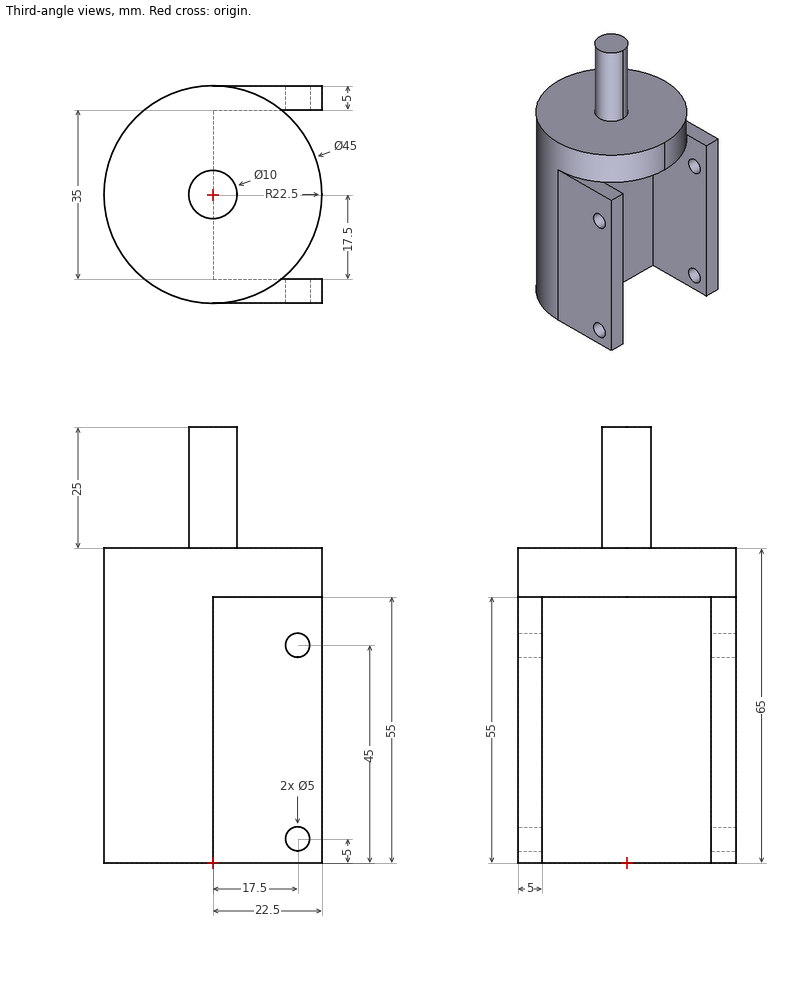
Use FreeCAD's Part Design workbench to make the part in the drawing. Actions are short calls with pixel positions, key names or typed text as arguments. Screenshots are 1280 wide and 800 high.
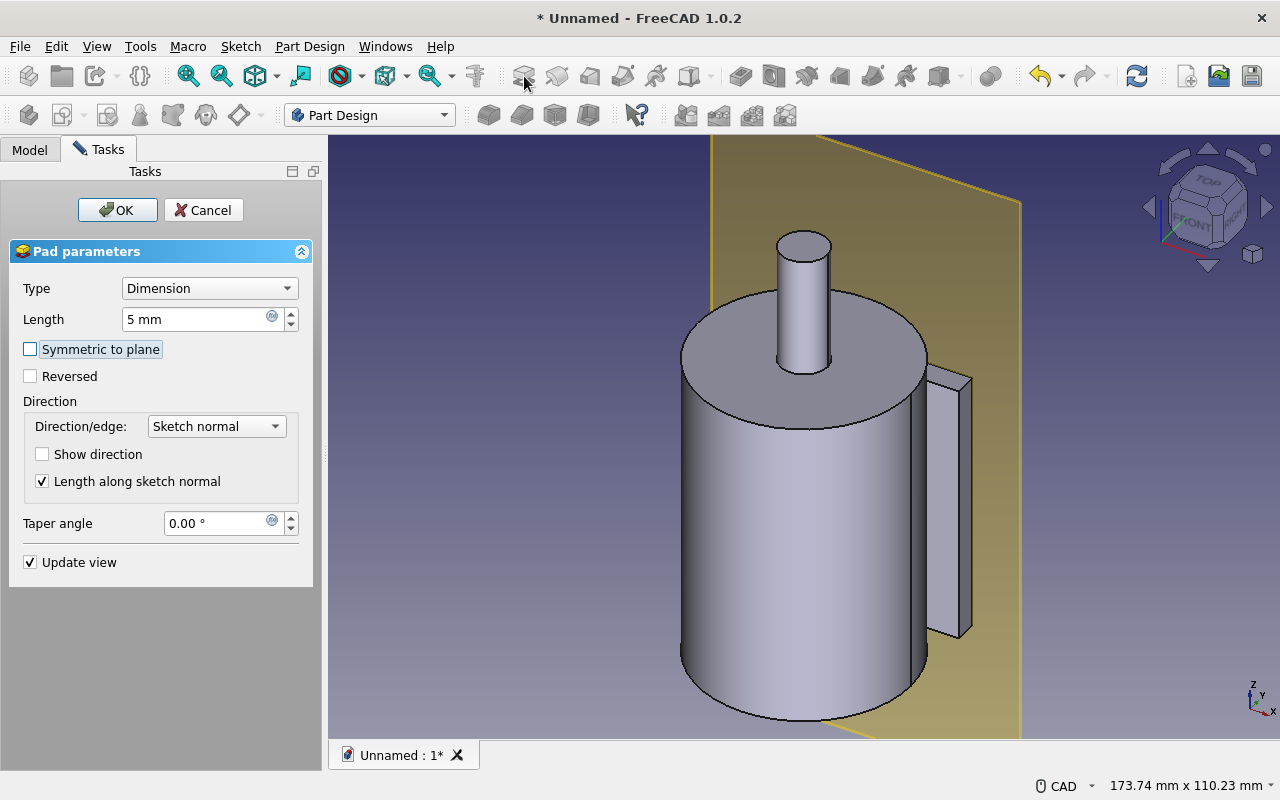
click(118, 210)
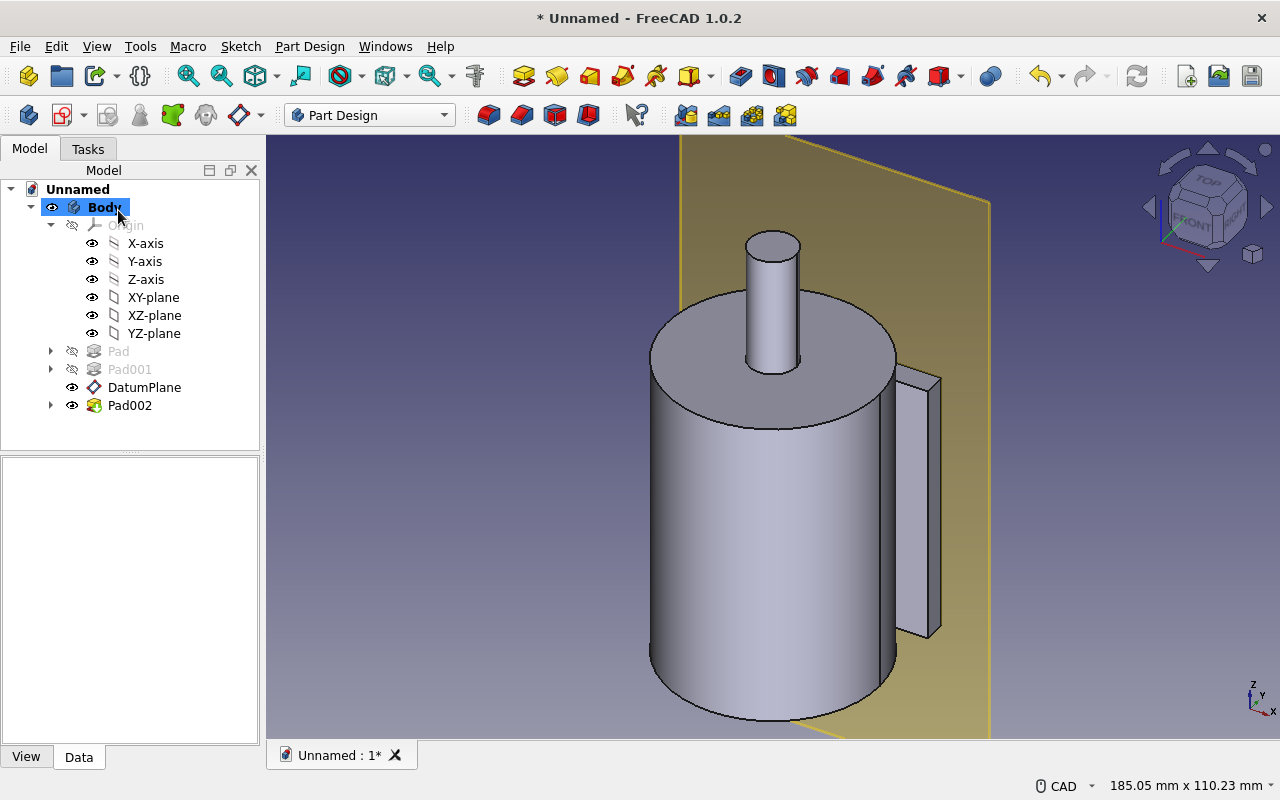
click(117, 387)
key(space)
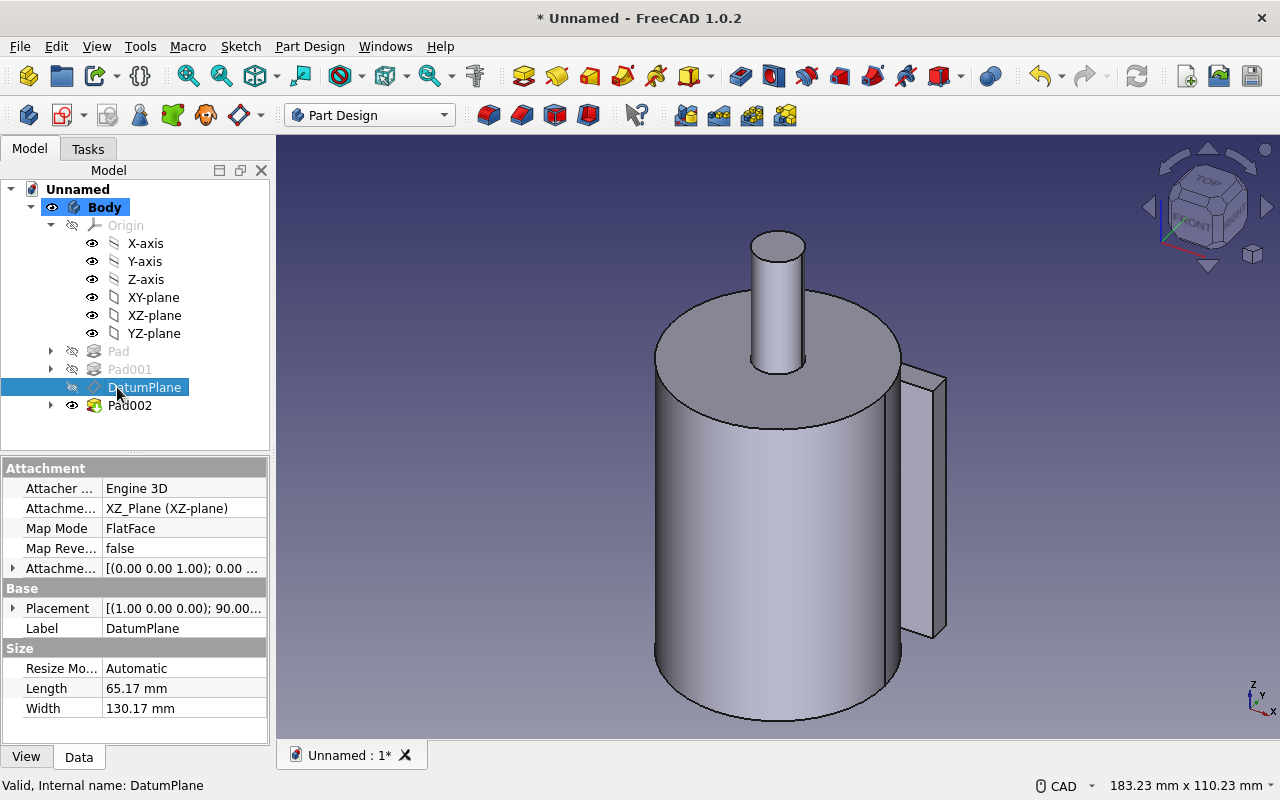
click(189, 76)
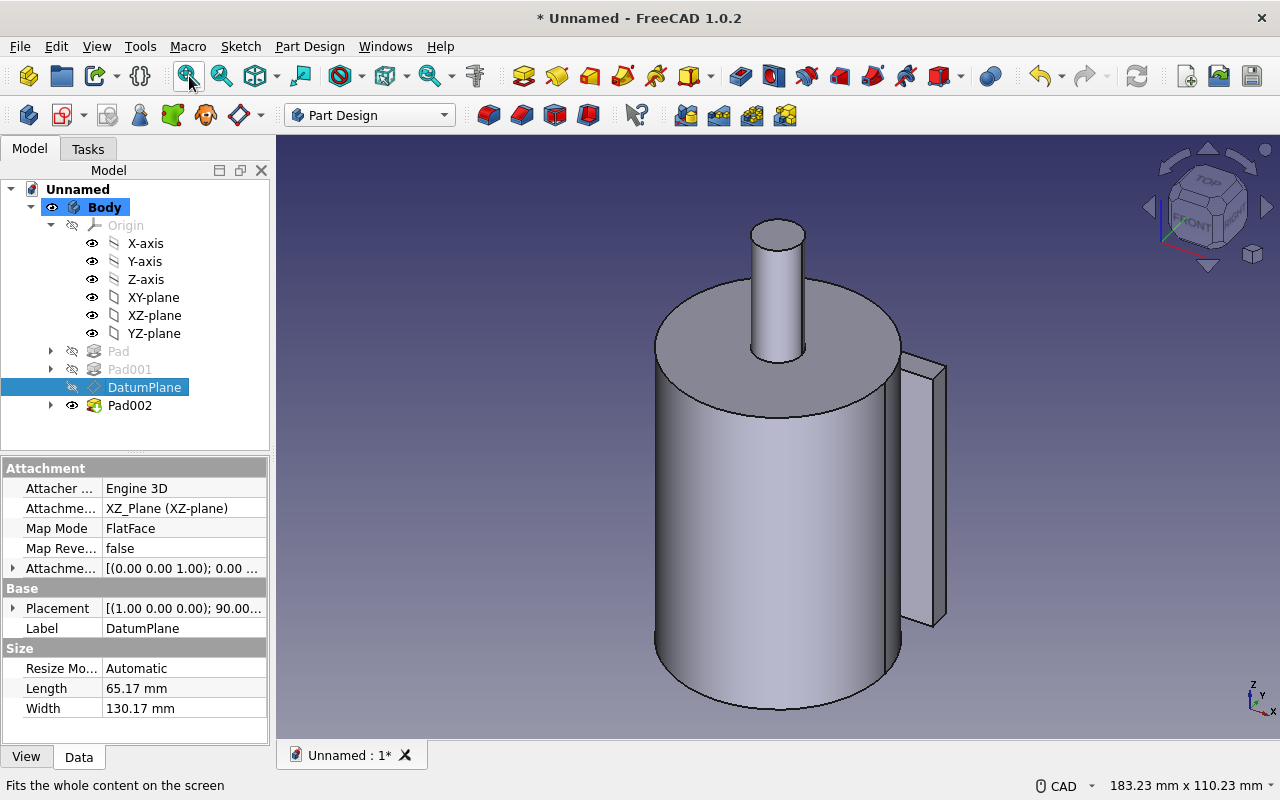
click(137, 315)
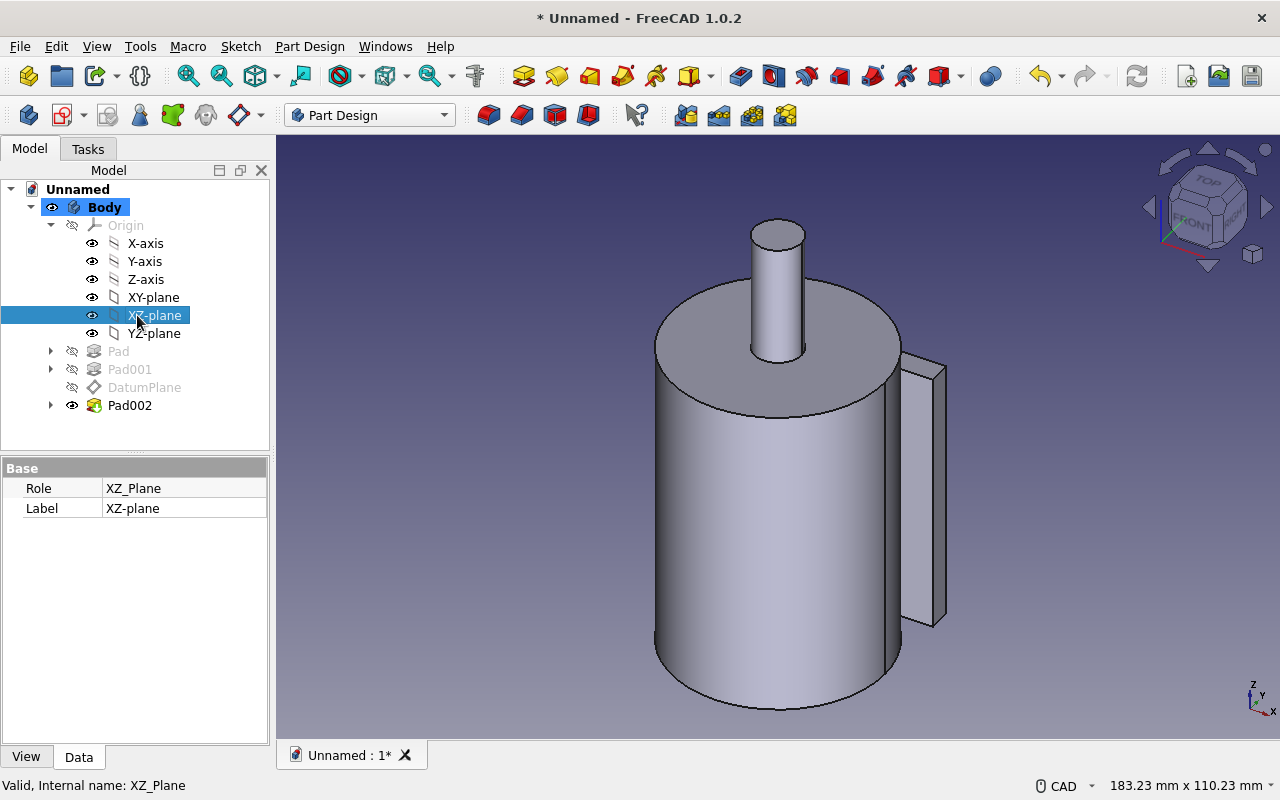
click(238, 116)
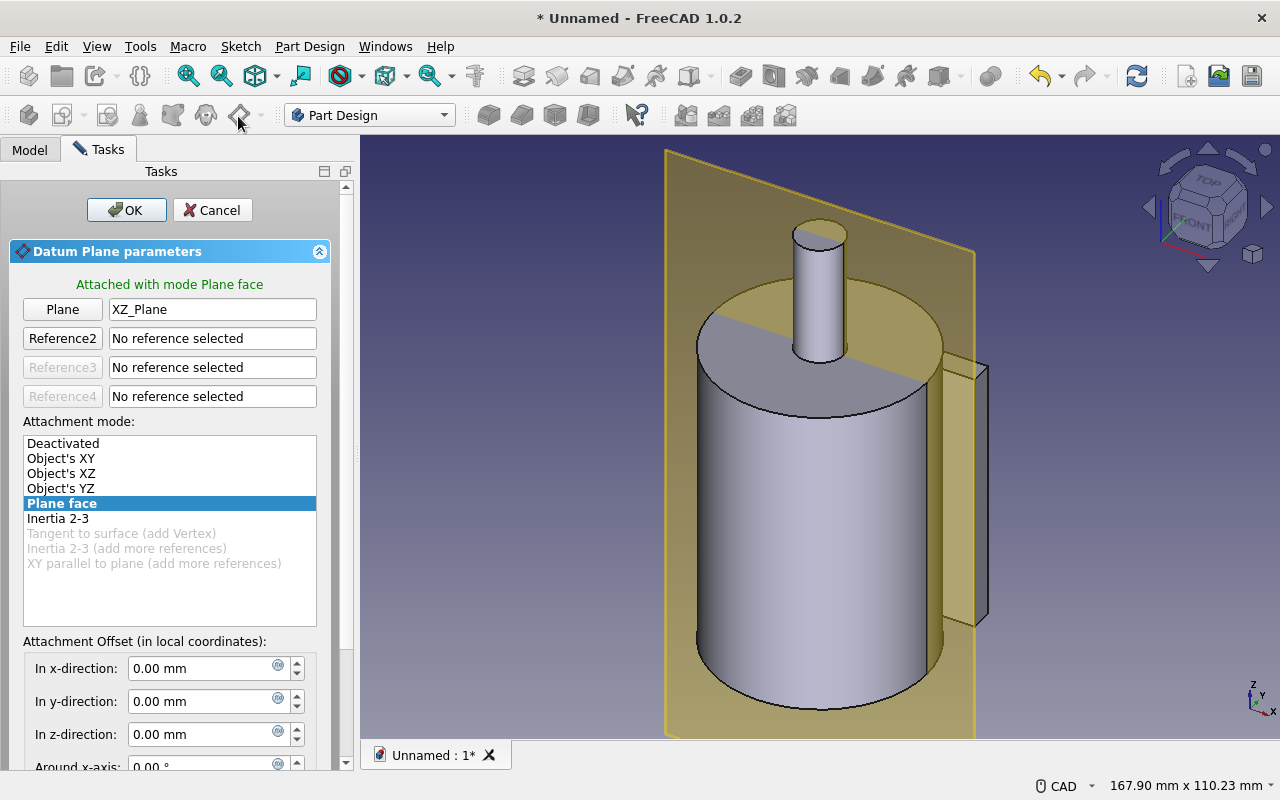
triple_click(210, 734)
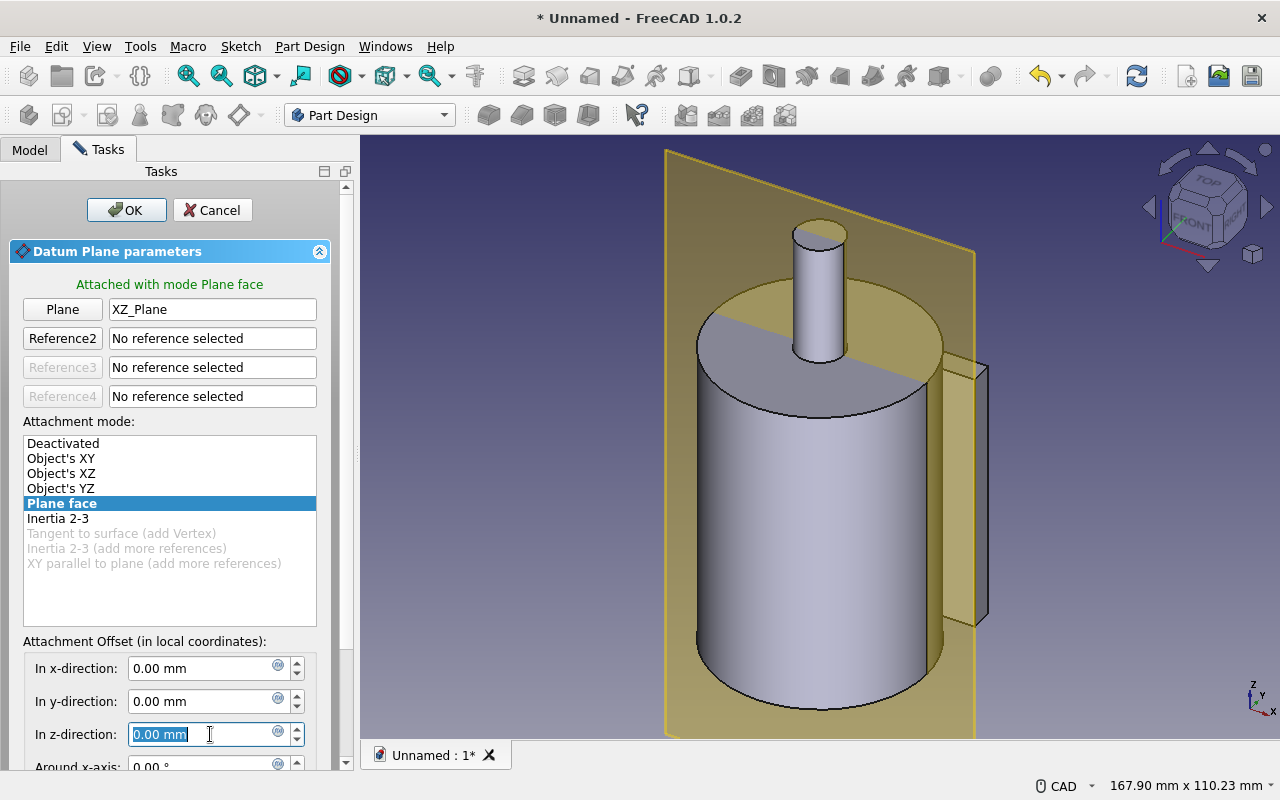
text(22.5)
key(Tab)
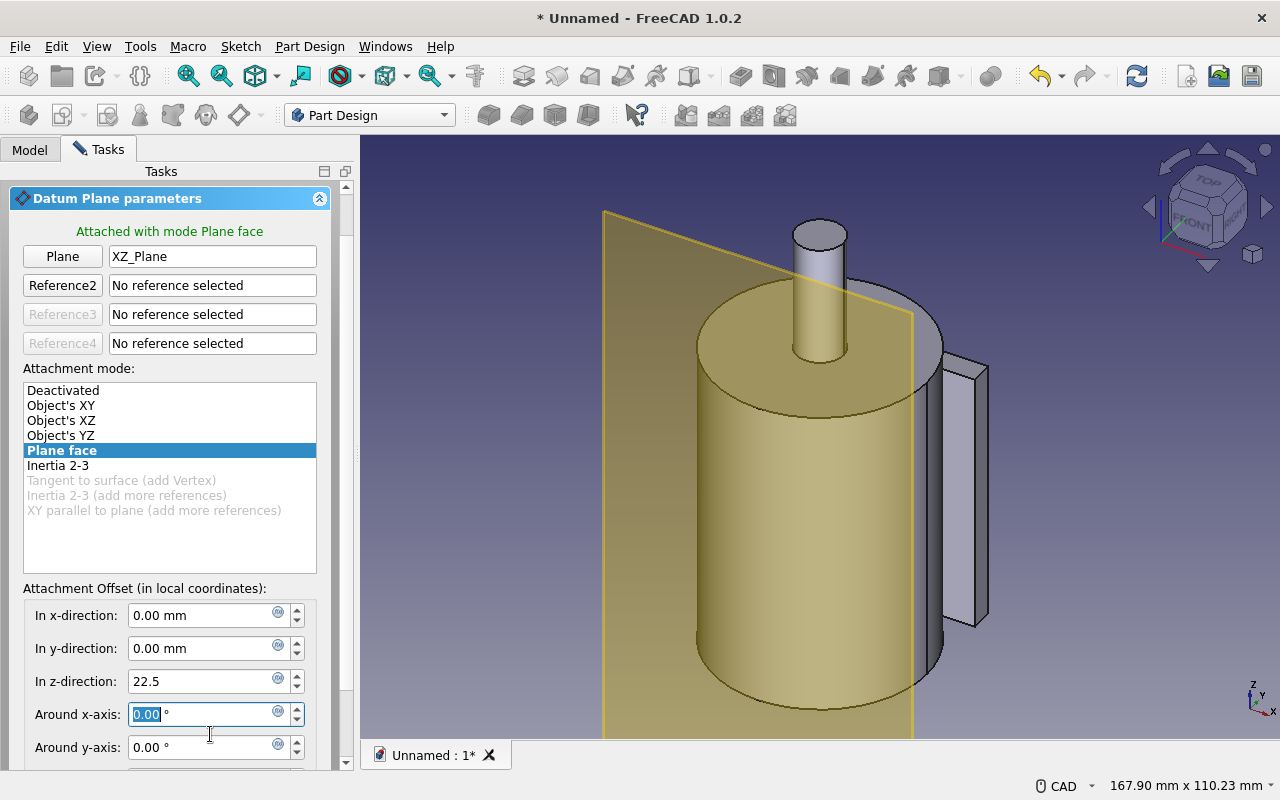
scroll(346, 476, up, 2)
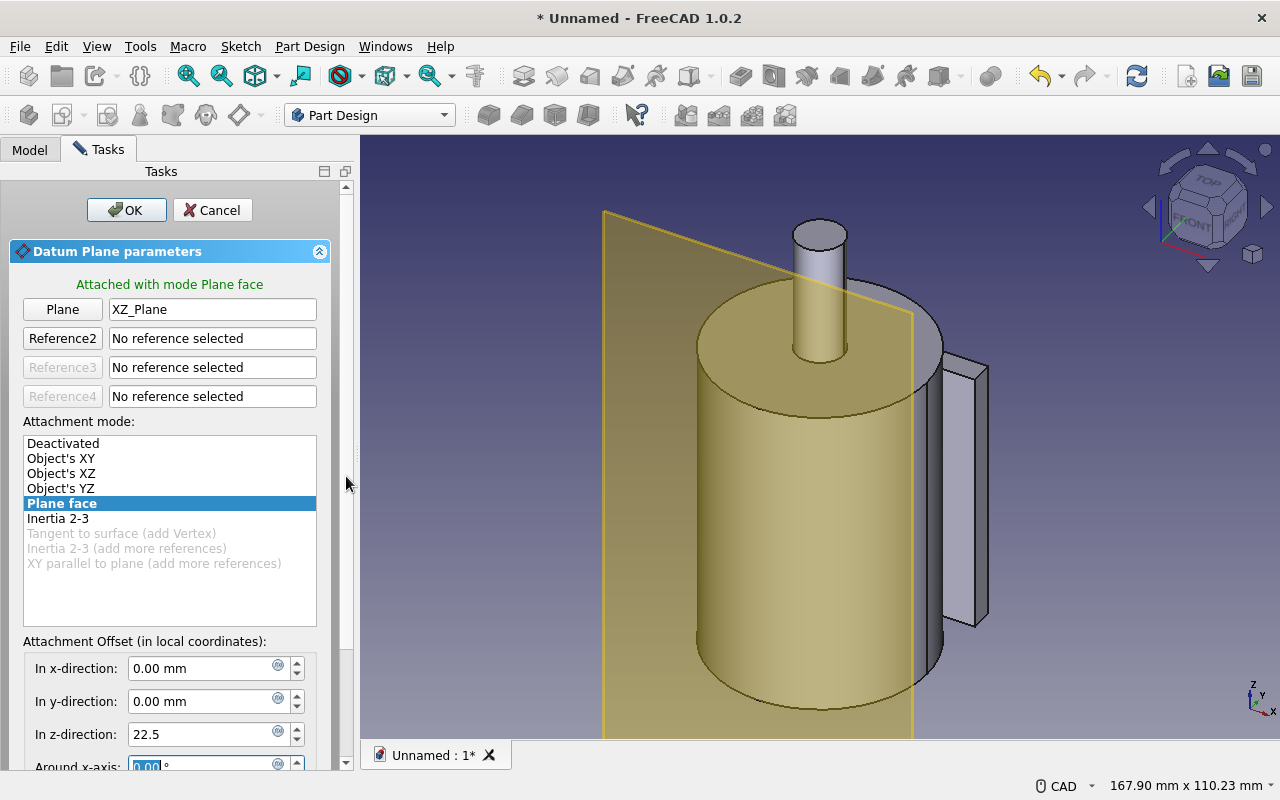
click(127, 210)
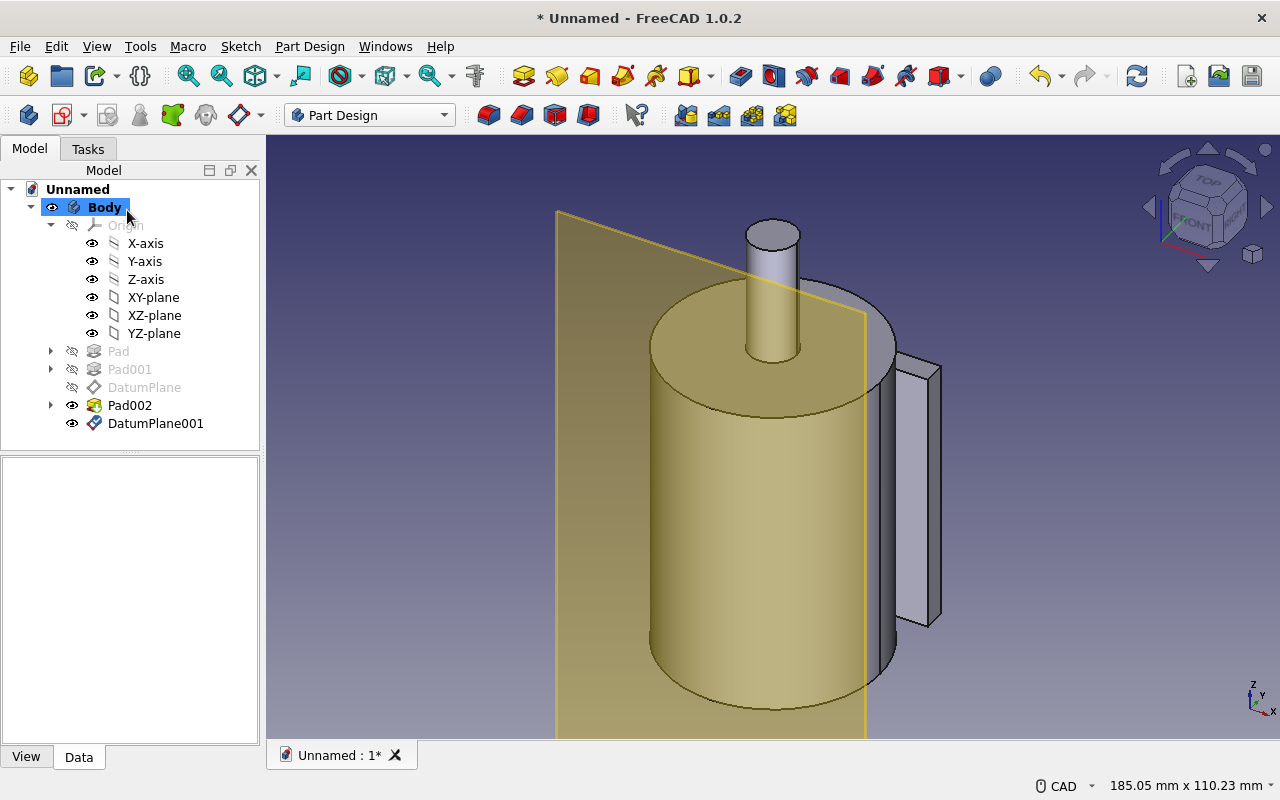
click(117, 423)